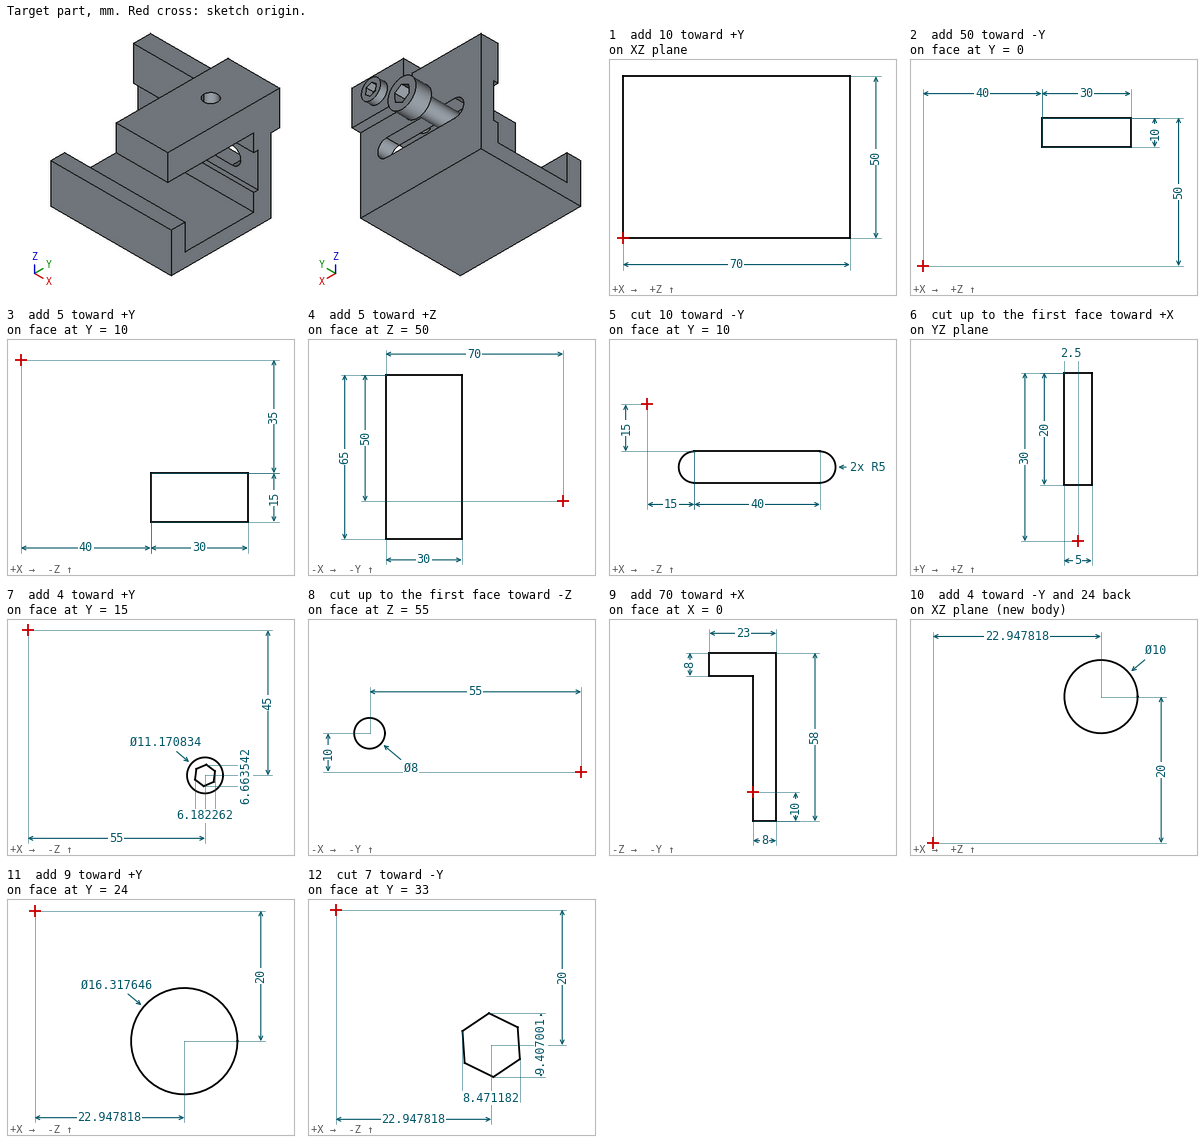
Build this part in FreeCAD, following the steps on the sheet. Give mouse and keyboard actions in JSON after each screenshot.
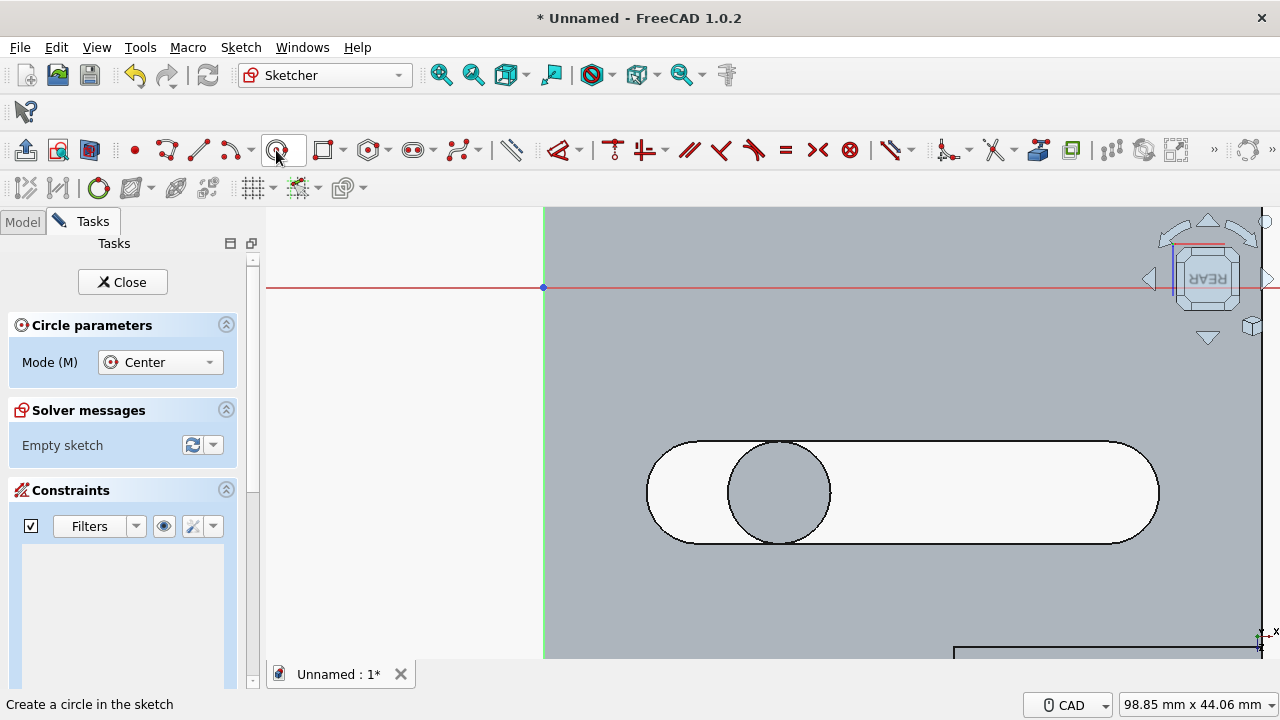
{"action": "left_click", "coordinate": [779, 493]}
{"action": "left_click", "coordinate": [838, 433]}
{"action": "key", "text": "Escape"}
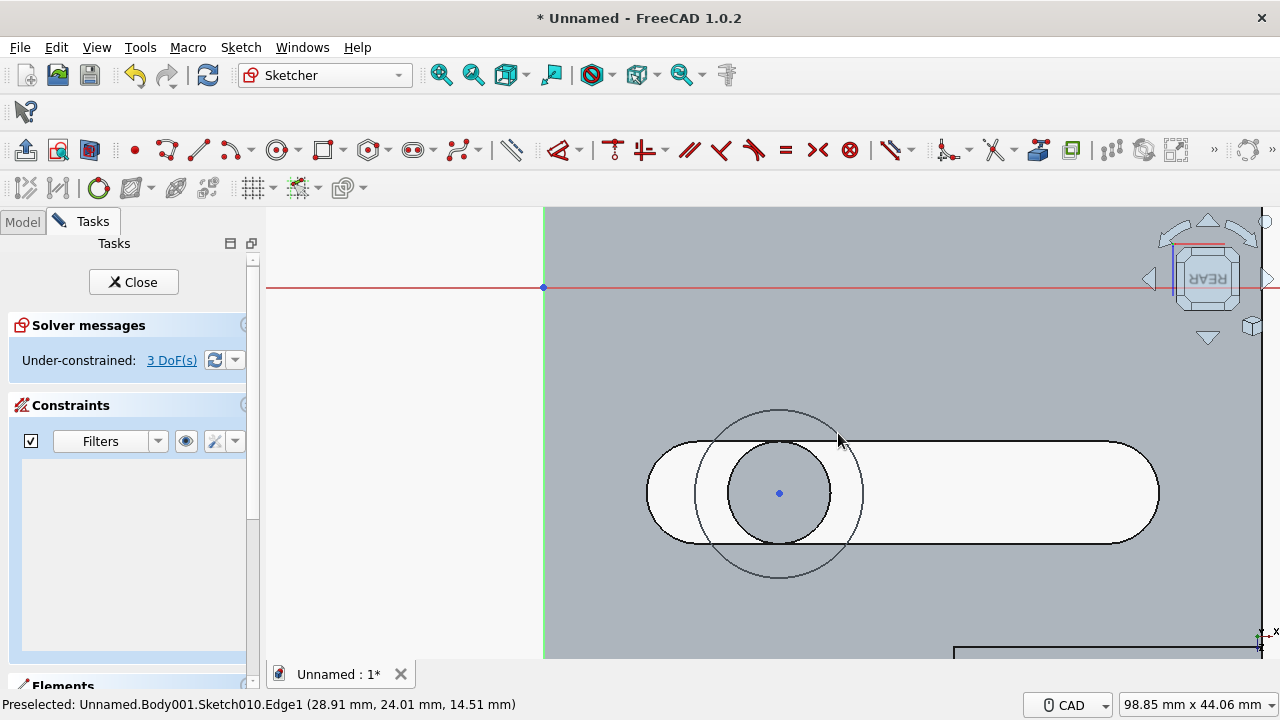
{"action": "left_click", "coordinate": [558, 150]}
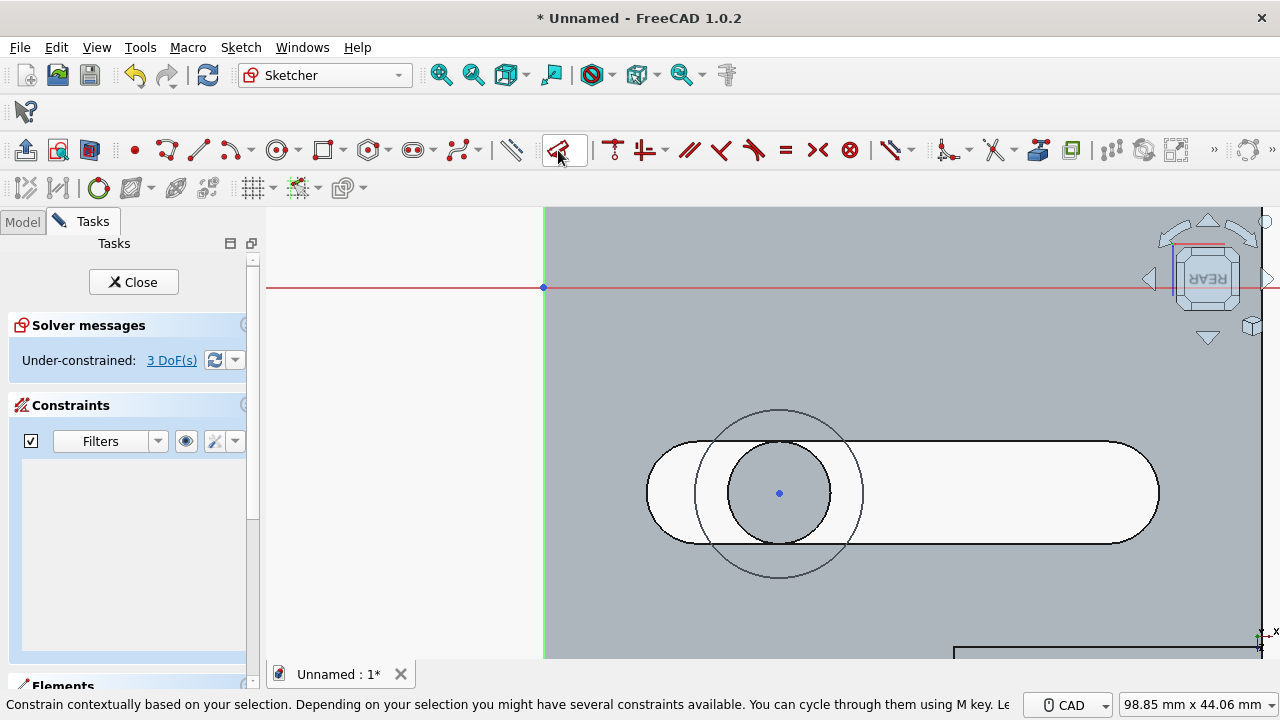
{"action": "left_click", "coordinate": [838, 434]}
{"action": "left_click", "coordinate": [860, 411]}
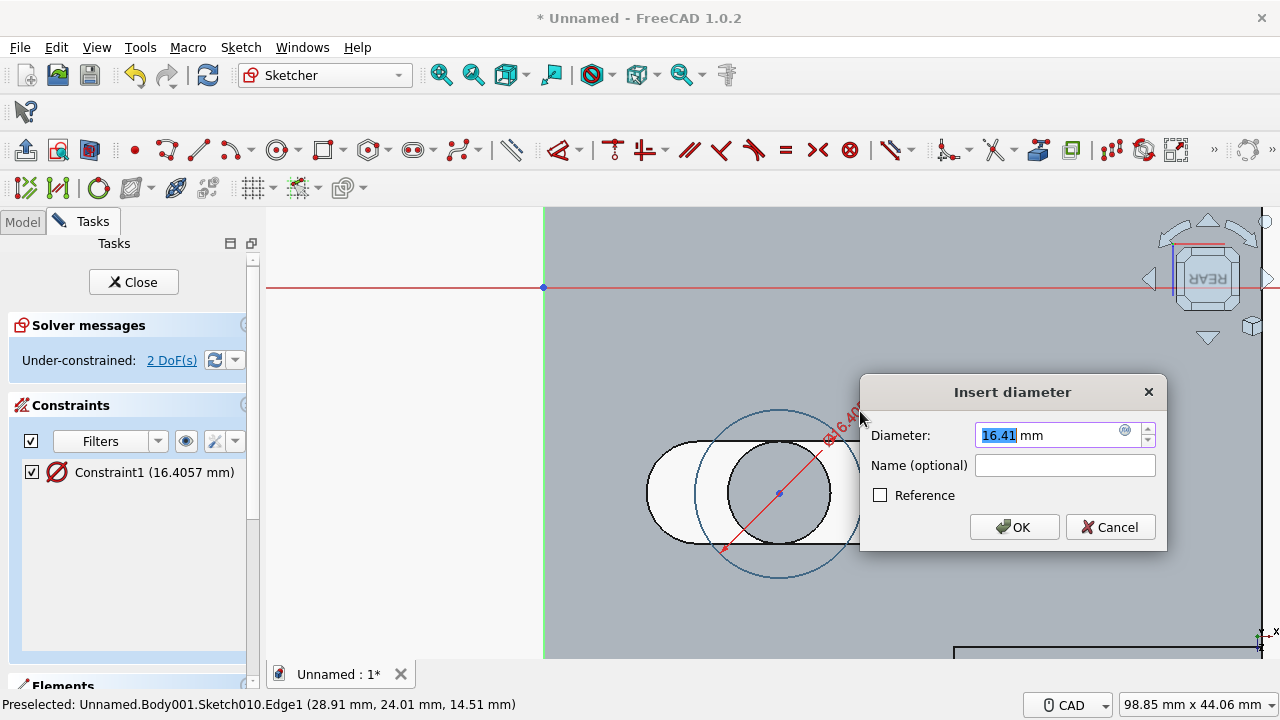
{"action": "type", "text": "16.317646"}
{"action": "key", "text": "Return"}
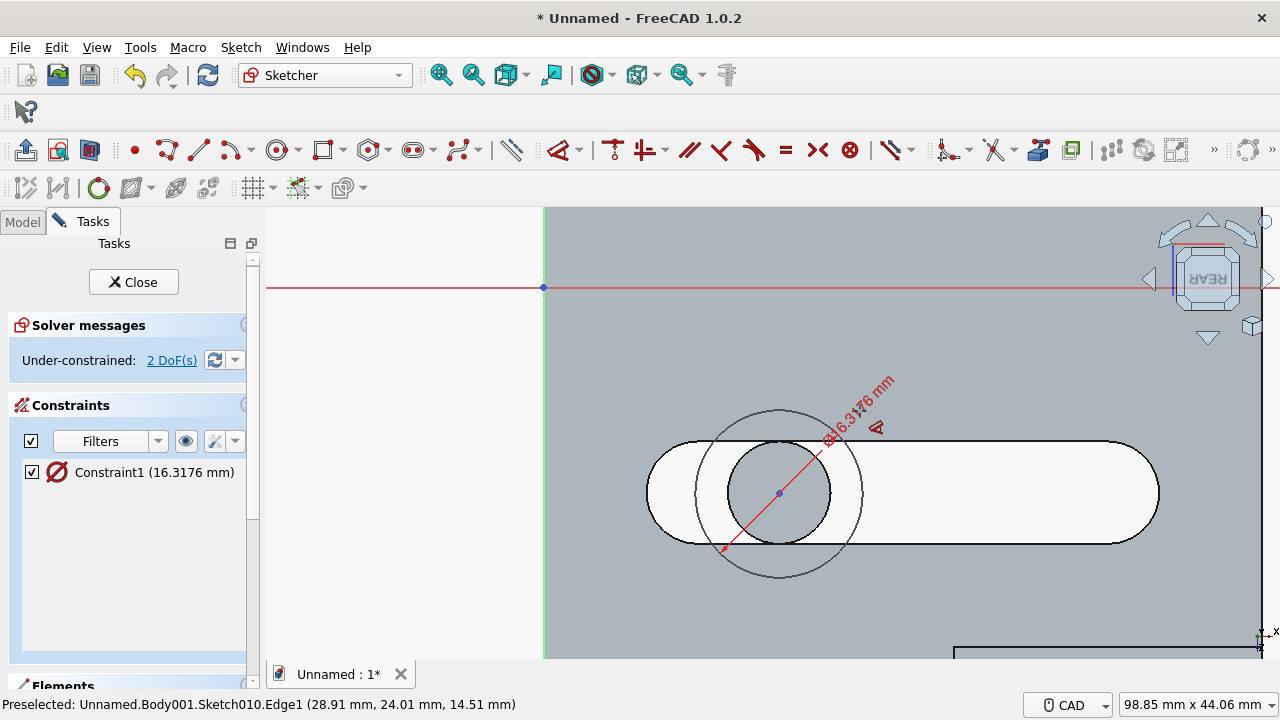
{"action": "left_click", "coordinate": [779, 494]}
{"action": "left_click", "coordinate": [510, 391]}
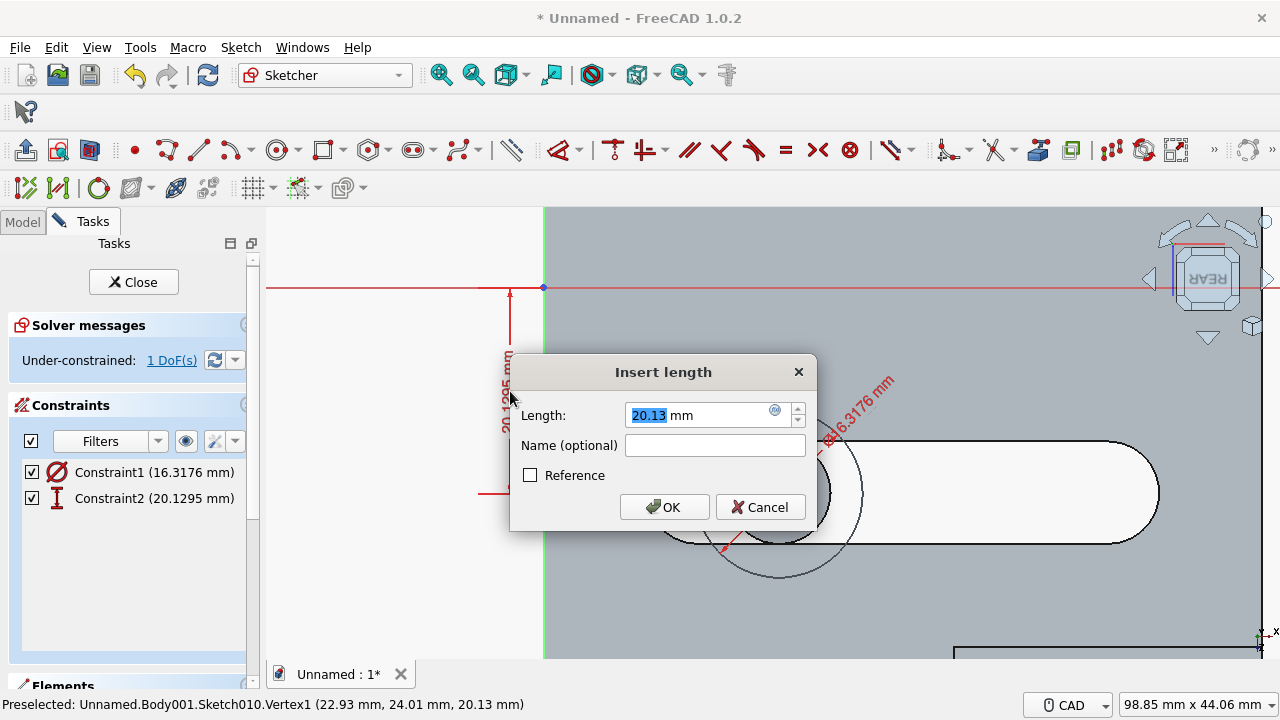
{"action": "type", "text": "20"}
{"action": "key", "text": "Return"}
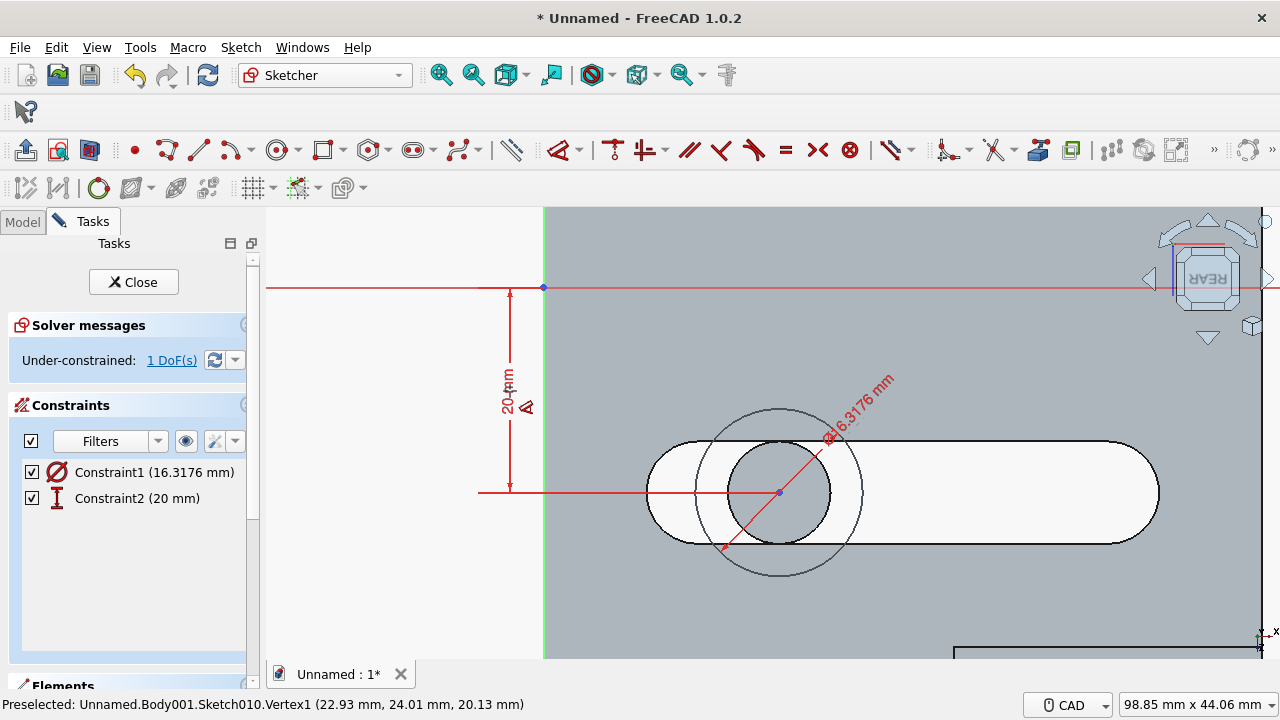
{"action": "left_click", "coordinate": [779, 493]}
{"action": "left_click", "coordinate": [661, 254]}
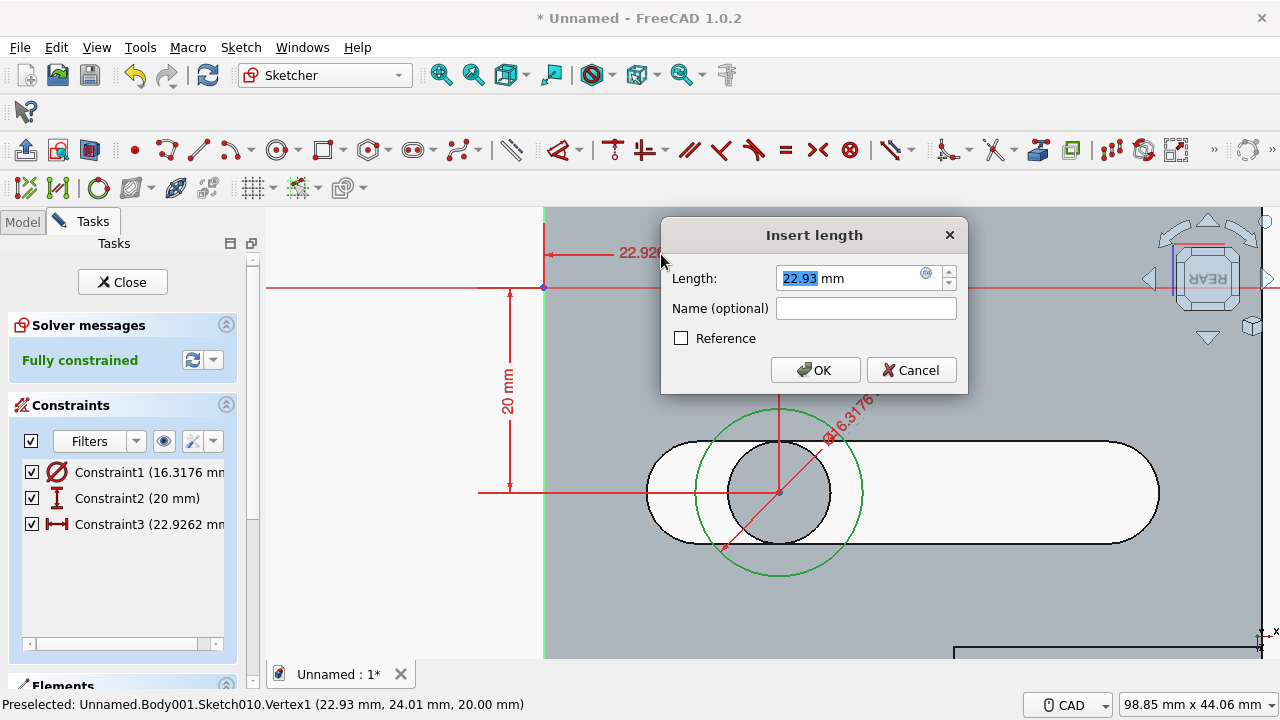
{"action": "type", "text": "22.947818"}
{"action": "key", "text": "Return"}
{"action": "key", "text": "Escape"}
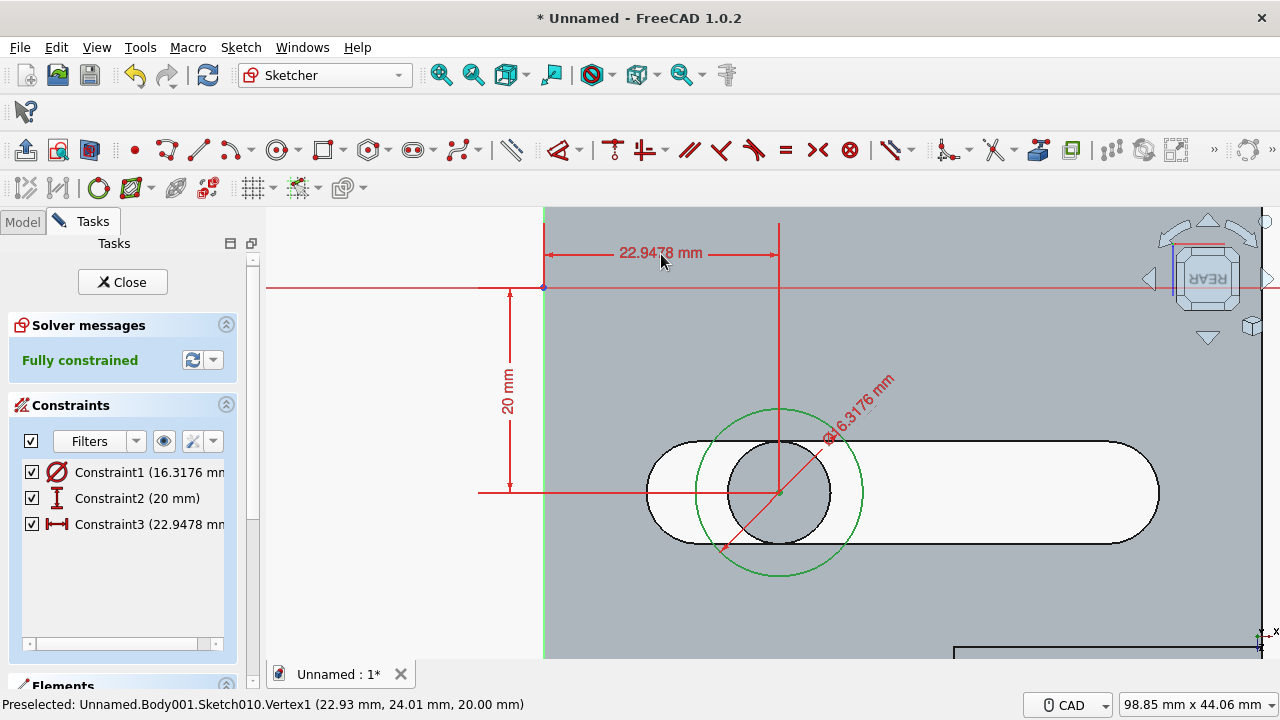
{"action": "left_click", "coordinate": [123, 282]}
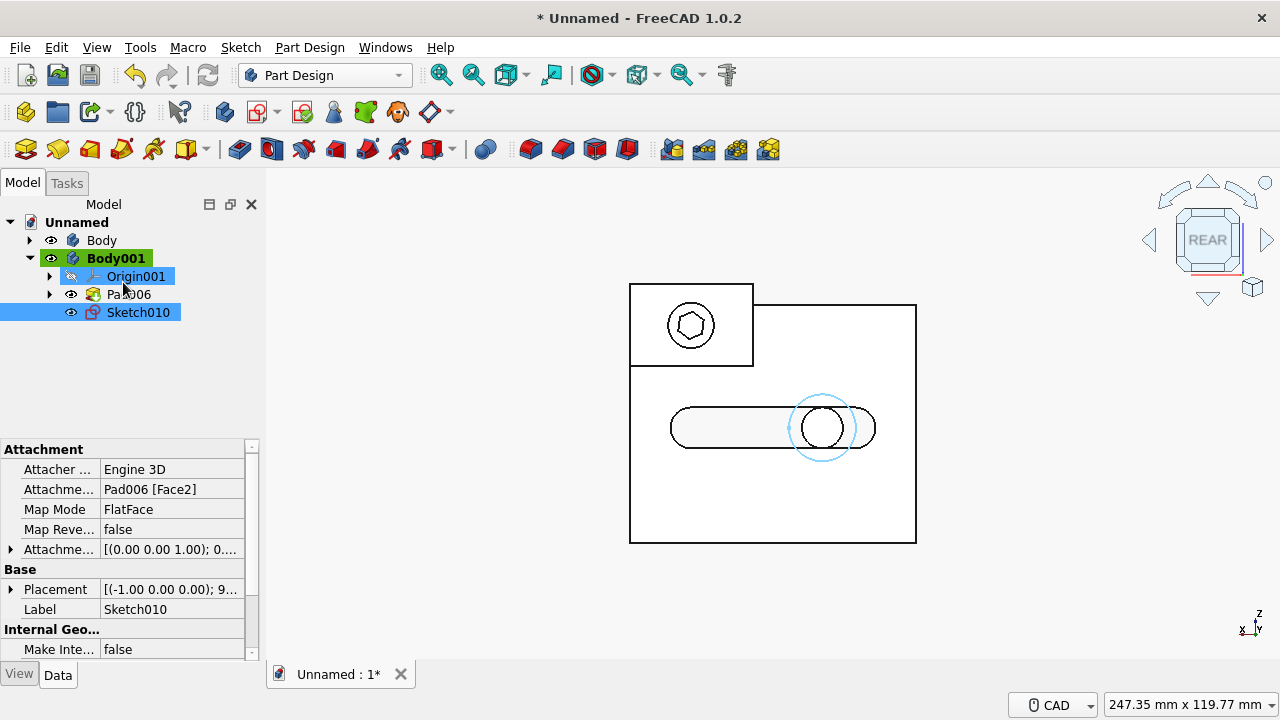
{"action": "left_click", "coordinate": [26, 150]}